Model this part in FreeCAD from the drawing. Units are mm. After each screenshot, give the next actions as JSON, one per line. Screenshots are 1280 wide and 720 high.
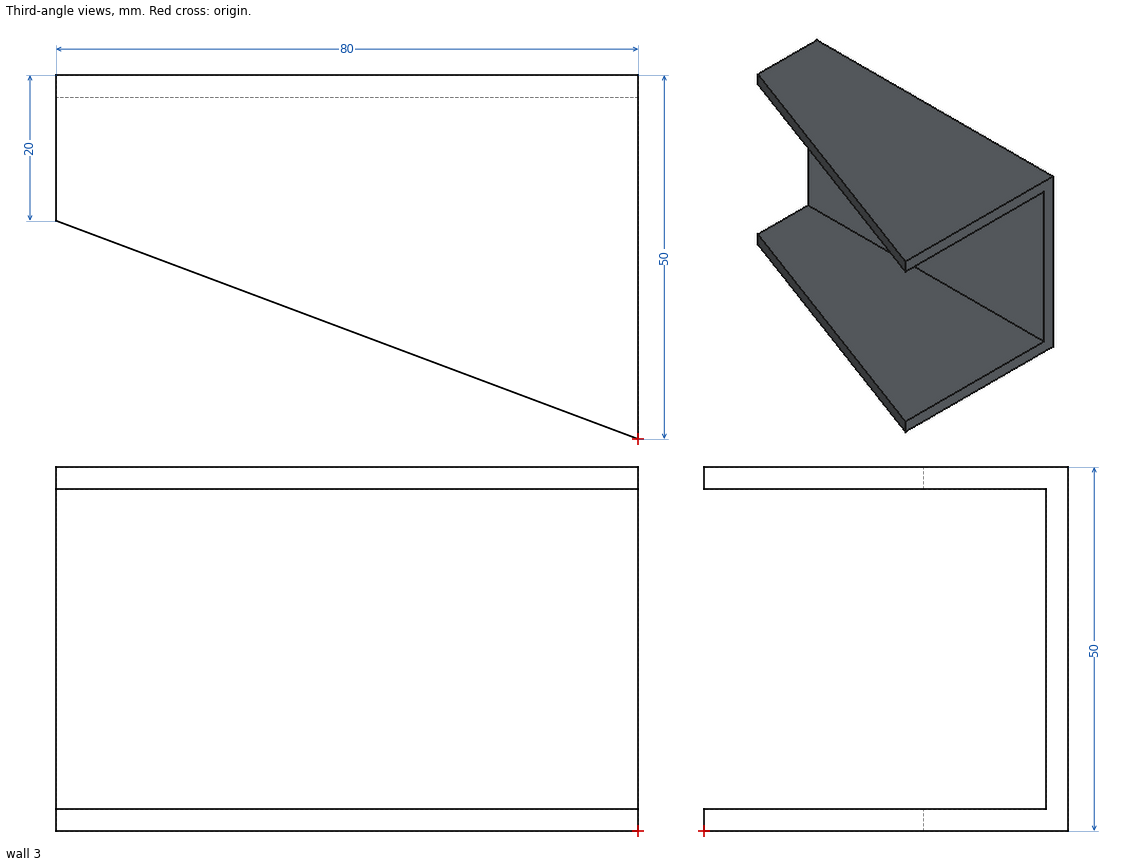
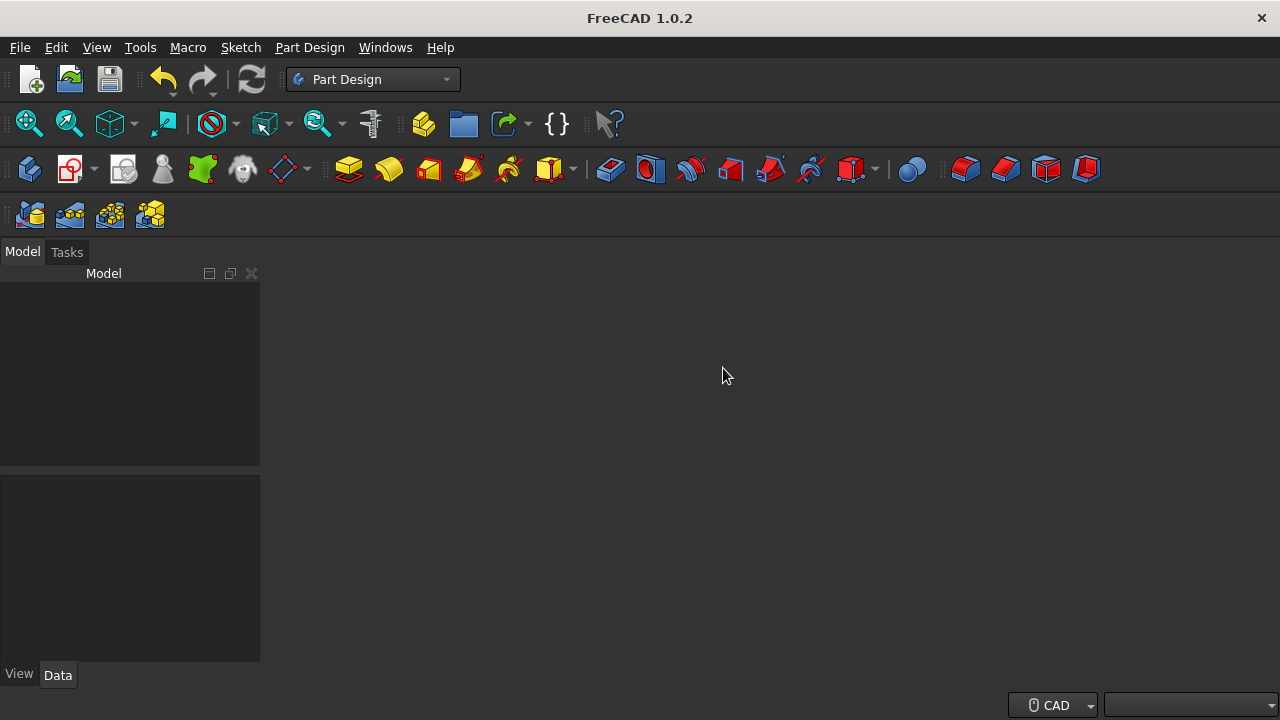
{"action": "key", "text": "ctrl+n"}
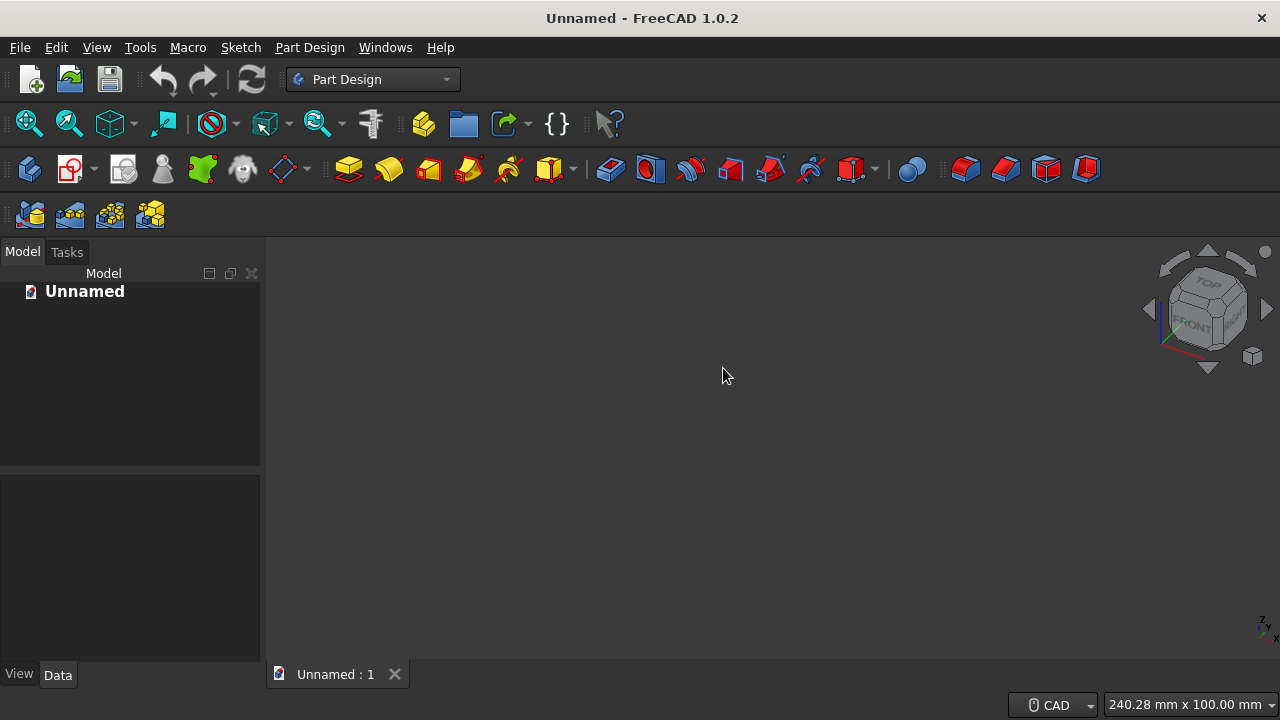
{"action": "left_click", "coordinate": [70, 170]}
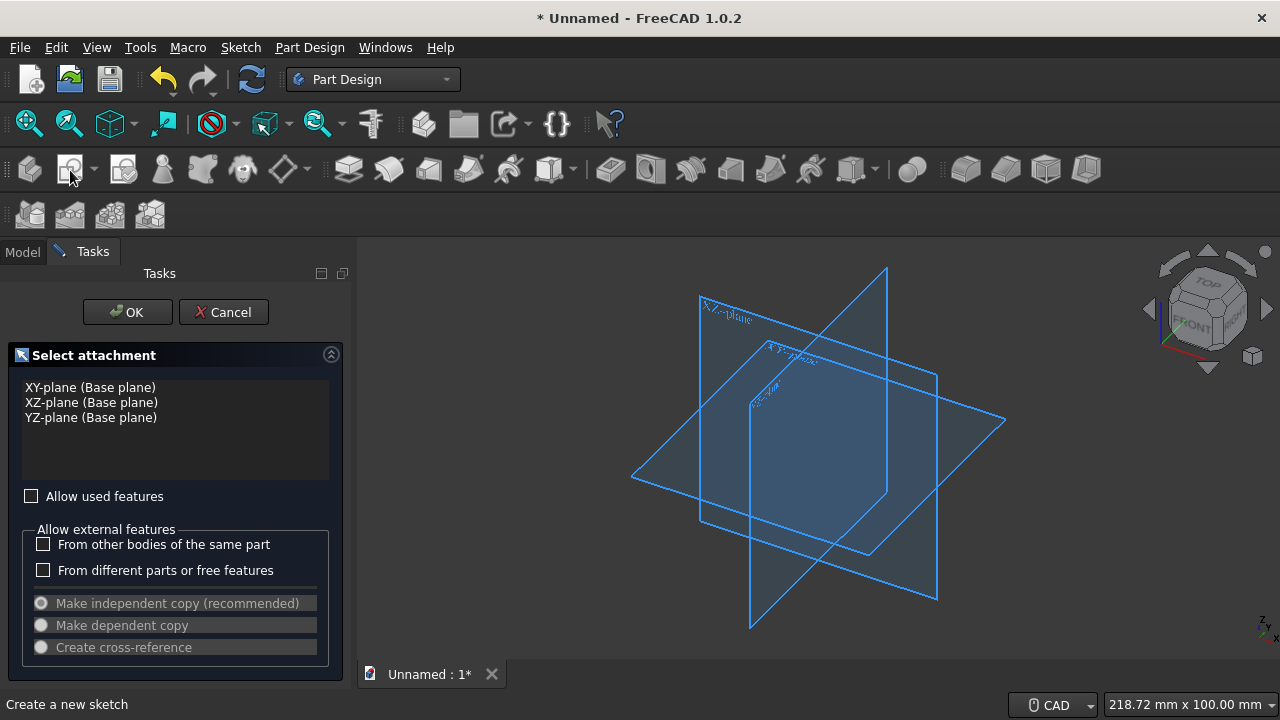
{"action": "left_click", "coordinate": [82, 388]}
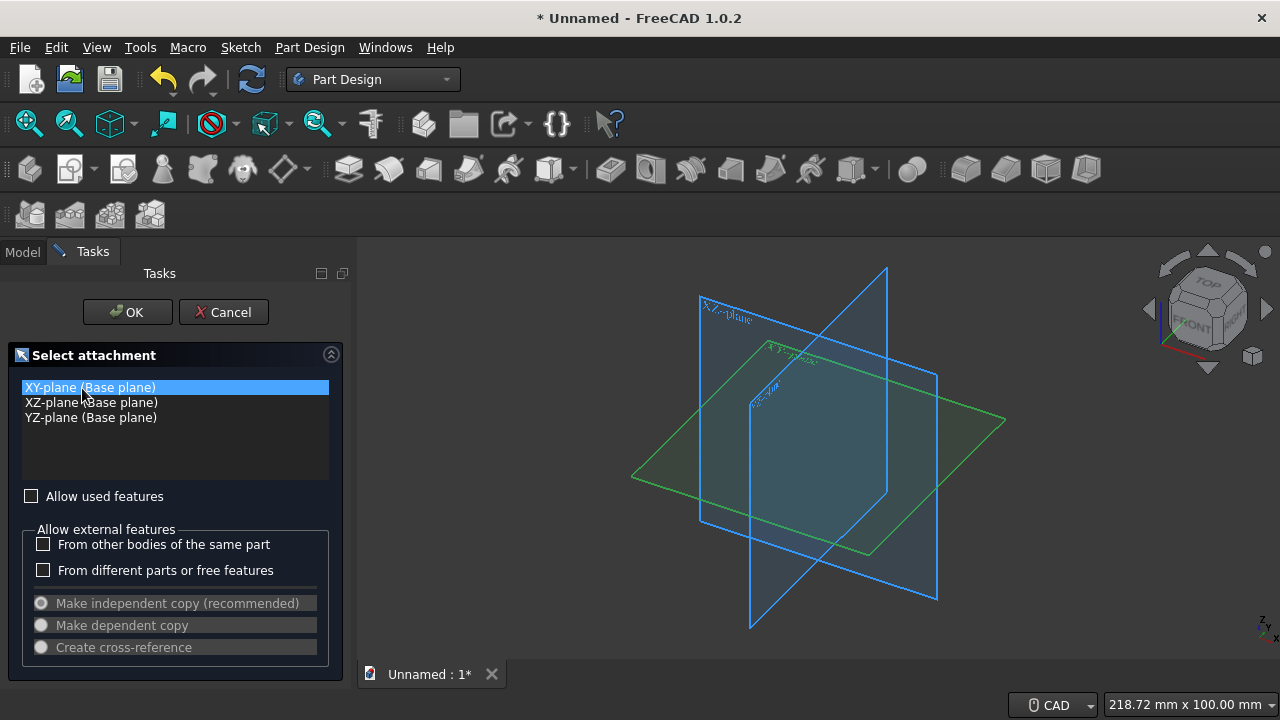
{"action": "left_click", "coordinate": [128, 312]}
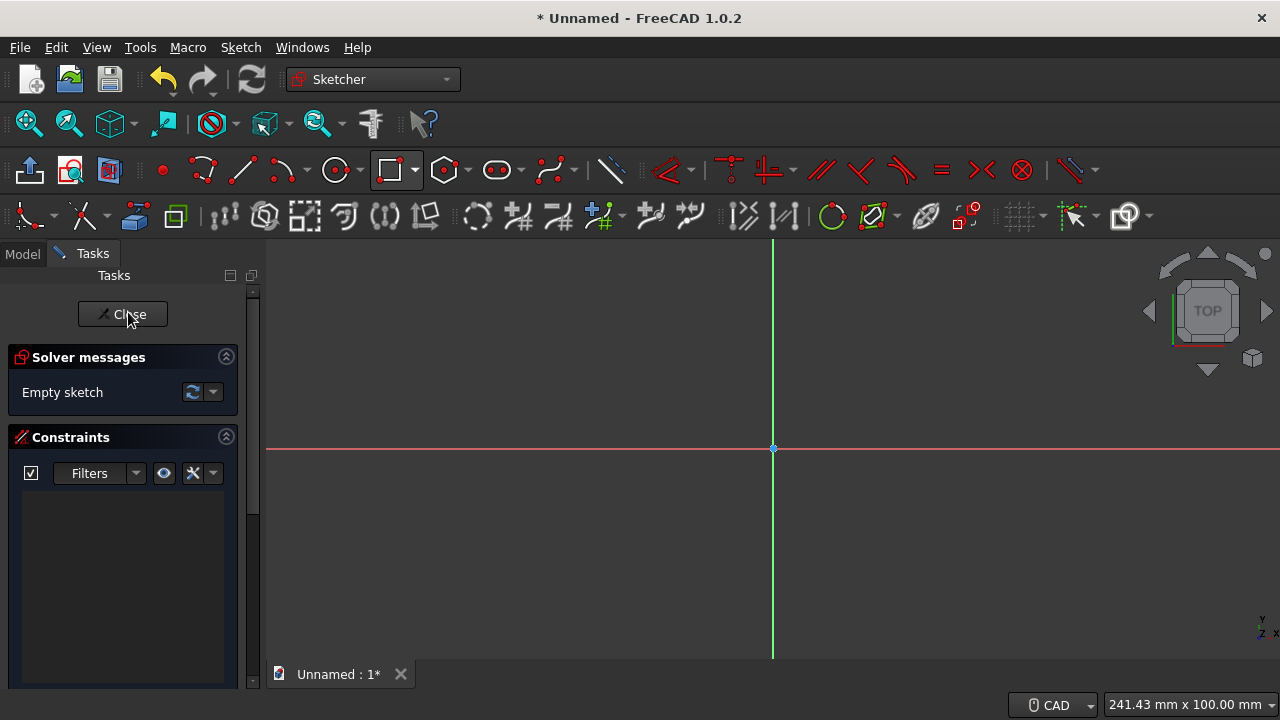
{"action": "scroll", "coordinate": [1115, 631], "scroll_direction": "down", "scroll_amount": 1}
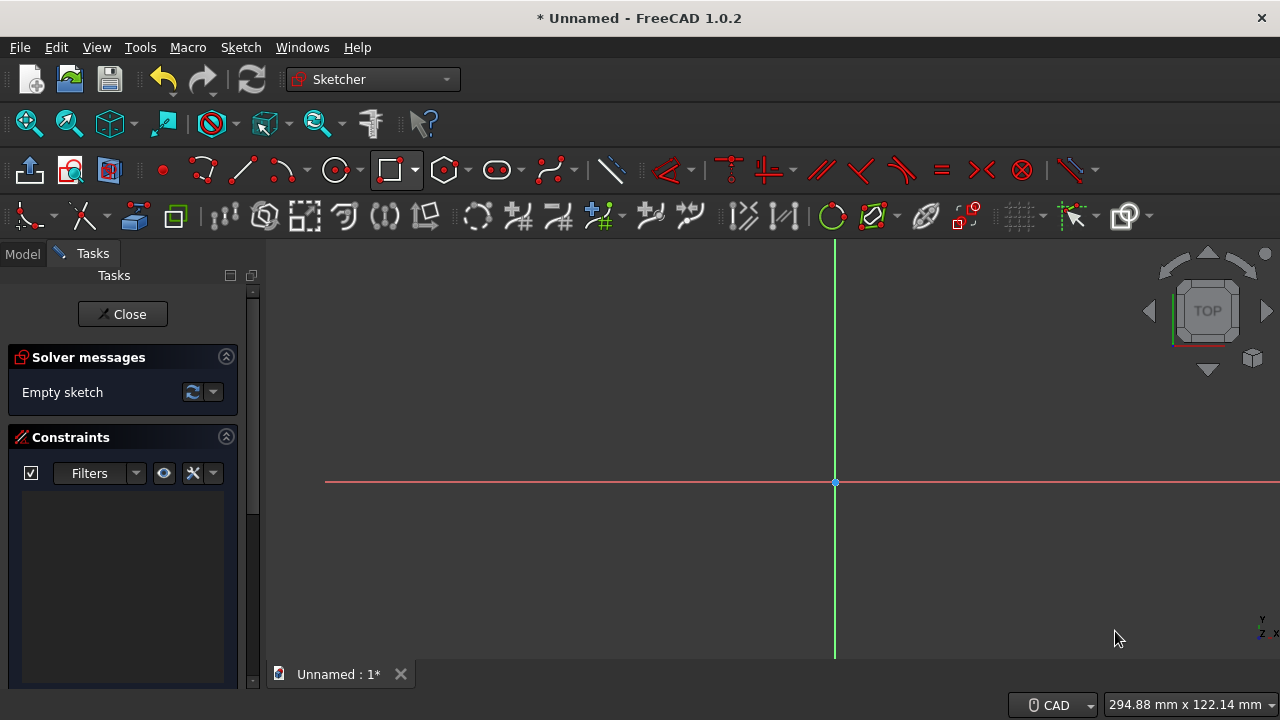
{"action": "scroll", "coordinate": [684, 289], "scroll_direction": "up", "scroll_amount": 2}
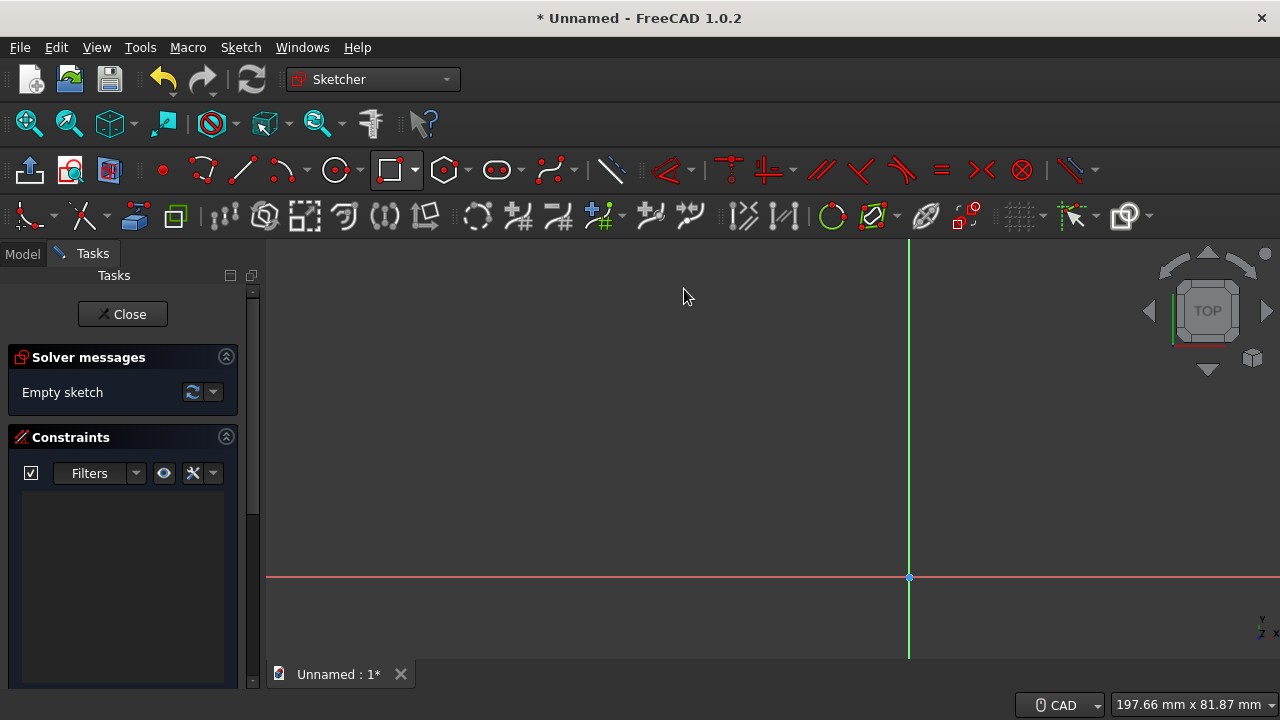
{"action": "key", "text": "g m"}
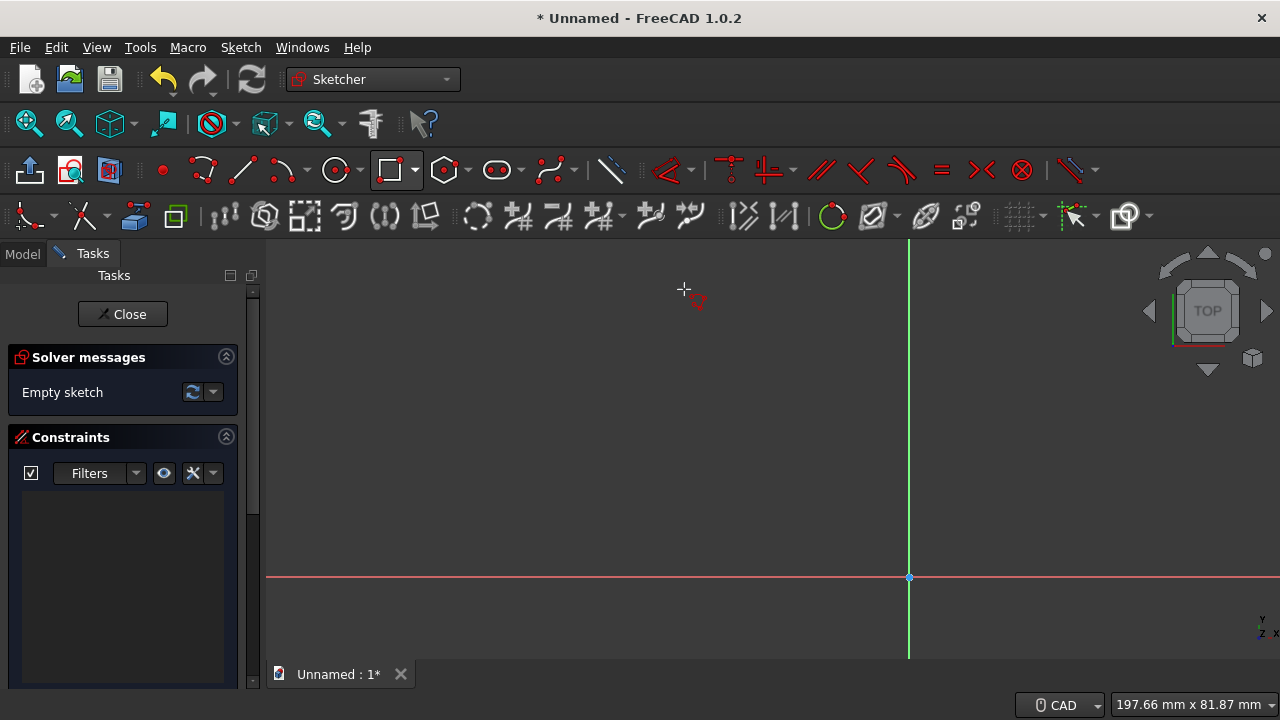
{"action": "left_click", "coordinate": [909, 577]}
{"action": "left_click", "coordinate": [900, 321]}
{"action": "left_click", "coordinate": [499, 321]}
{"action": "left_click", "coordinate": [499, 423]}
{"action": "left_click", "coordinate": [909, 577]}
{"action": "key", "text": "Escape"}
{"action": "key", "text": "Escape"}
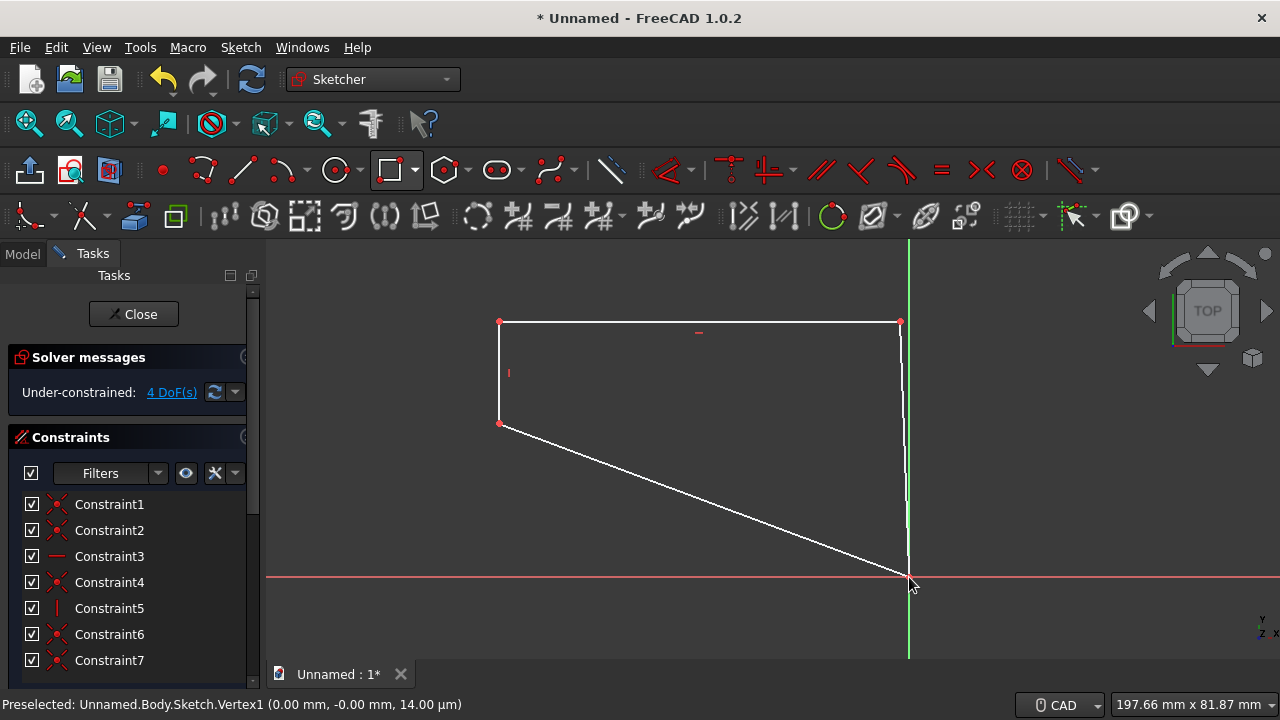
{"action": "left_click", "coordinate": [906, 501]}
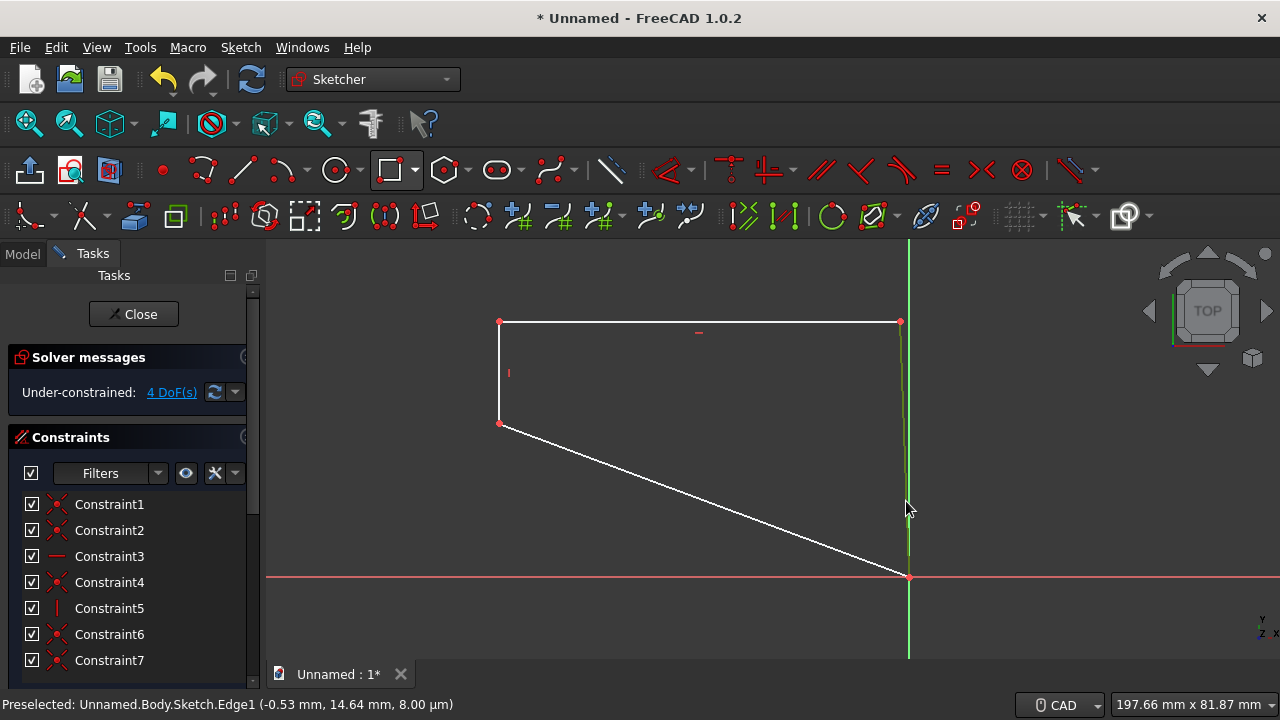
{"action": "key", "text": "v"}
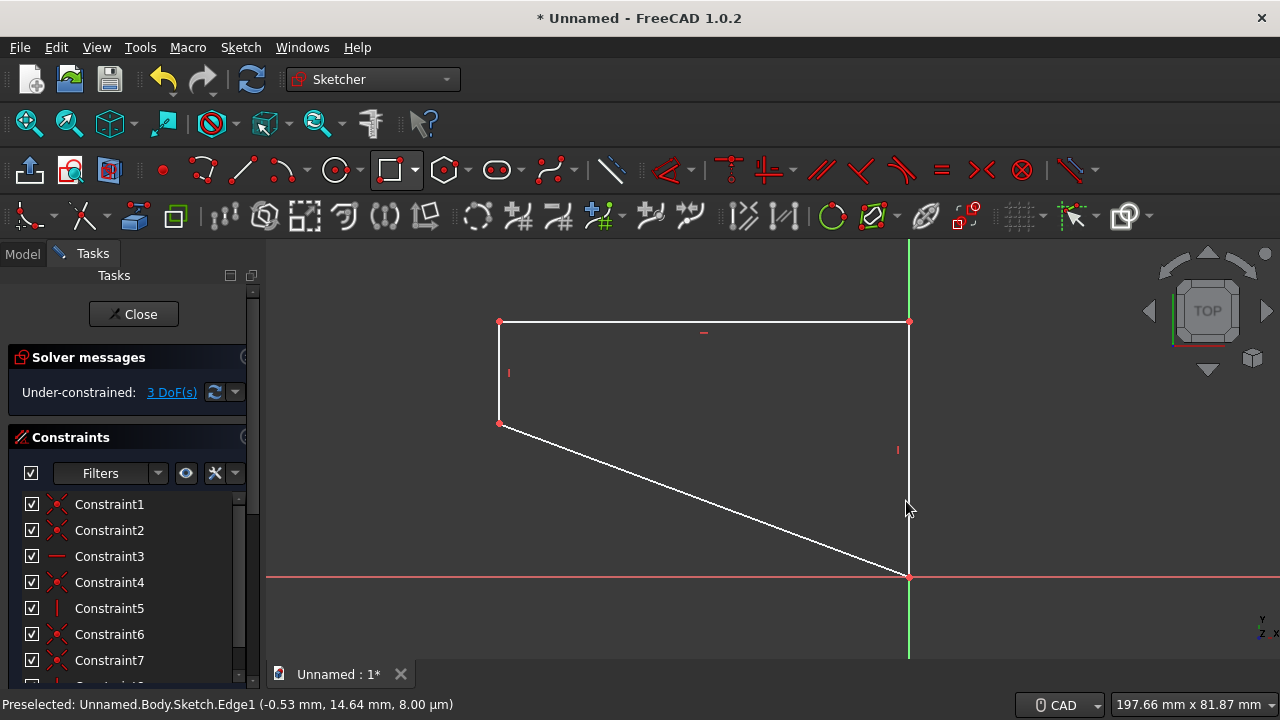
{"action": "key", "text": "d"}